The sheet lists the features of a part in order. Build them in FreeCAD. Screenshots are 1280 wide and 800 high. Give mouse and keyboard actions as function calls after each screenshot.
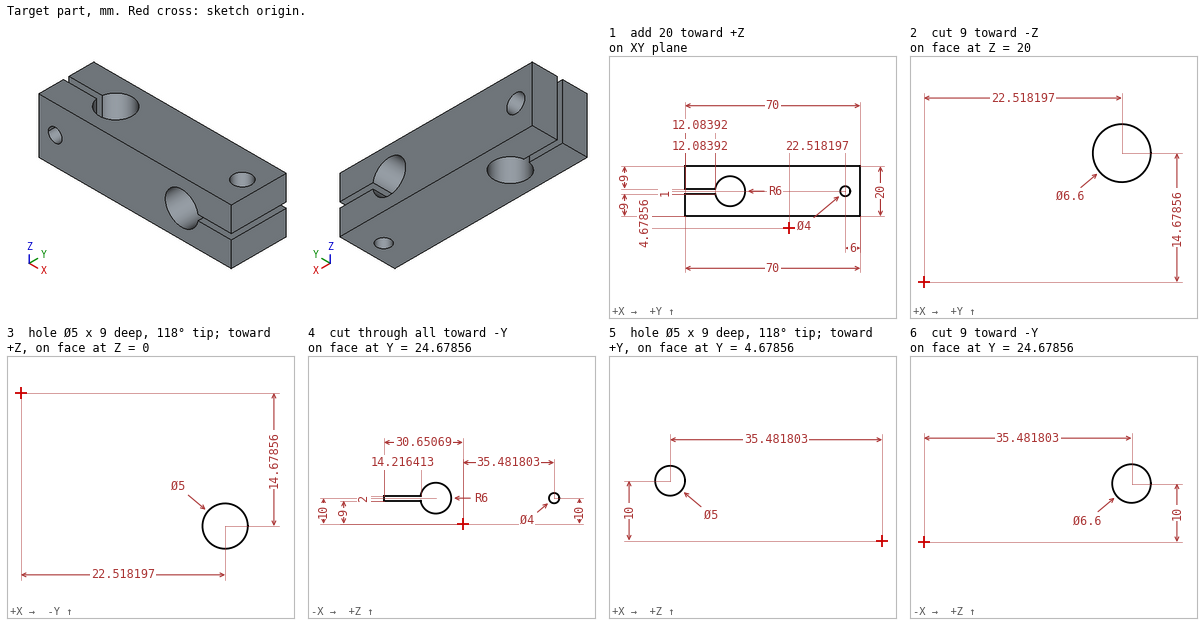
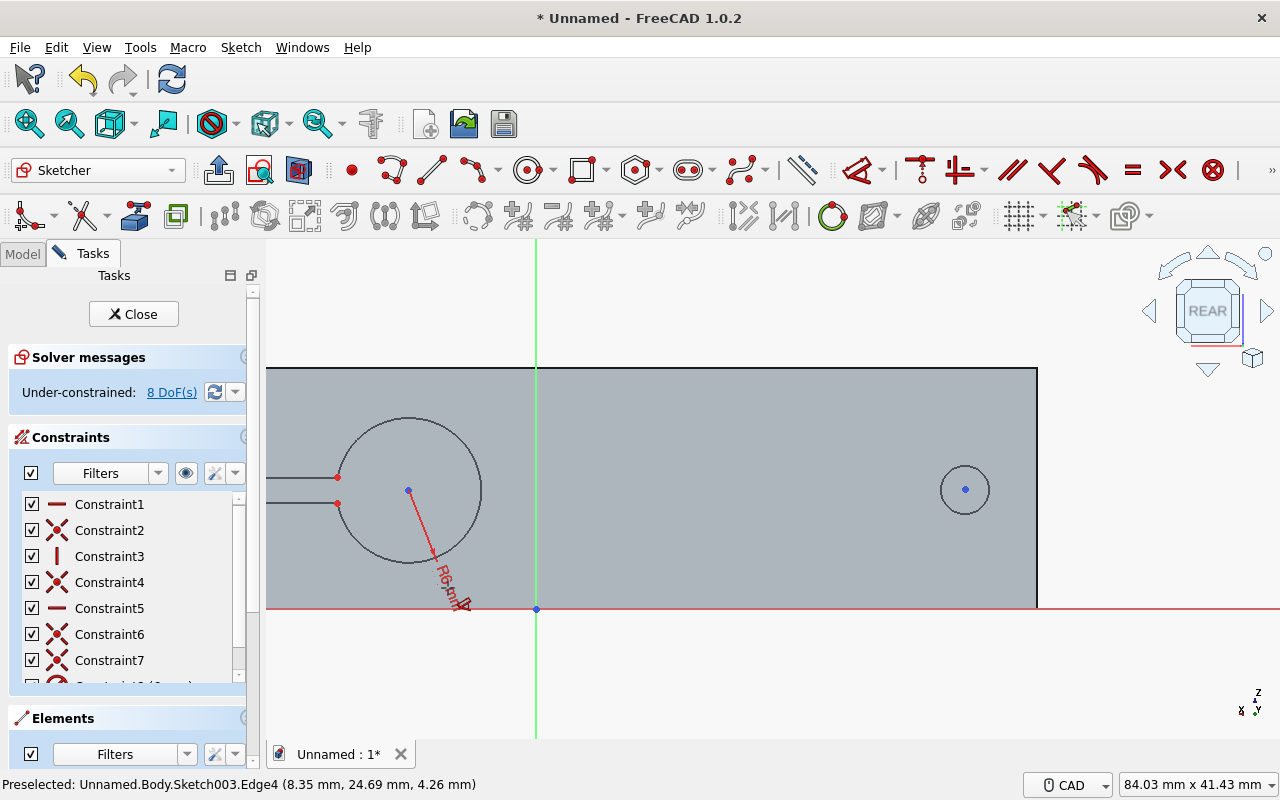
click(982, 473)
click(1005, 450)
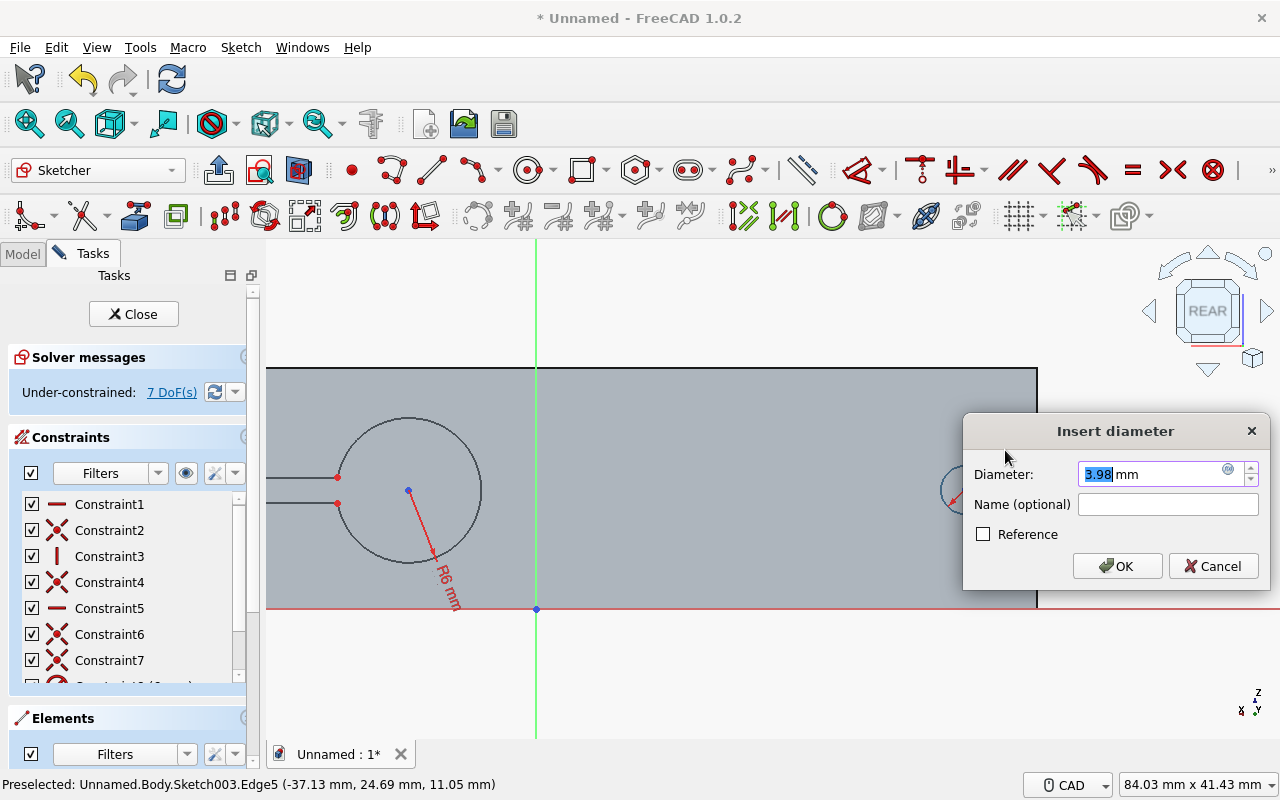
text(4)
key(Return)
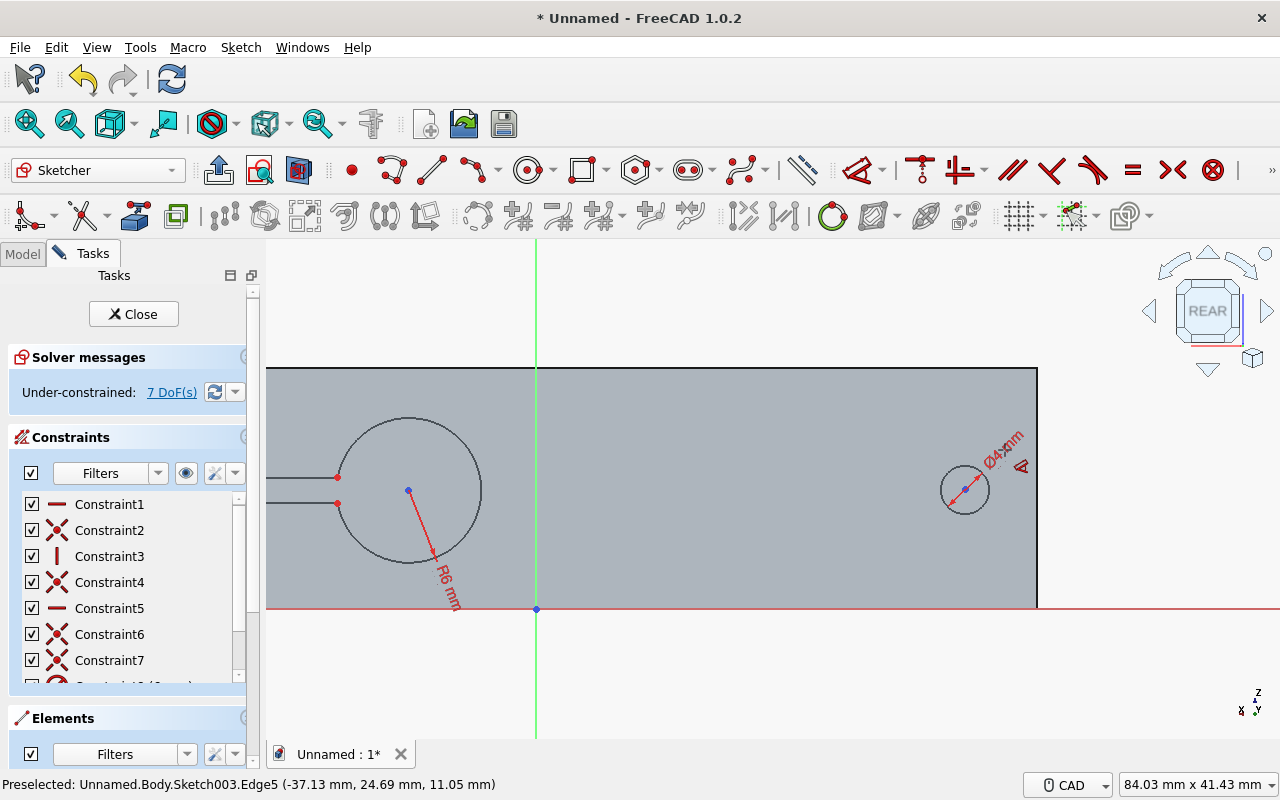
scroll(963, 392, down, 2)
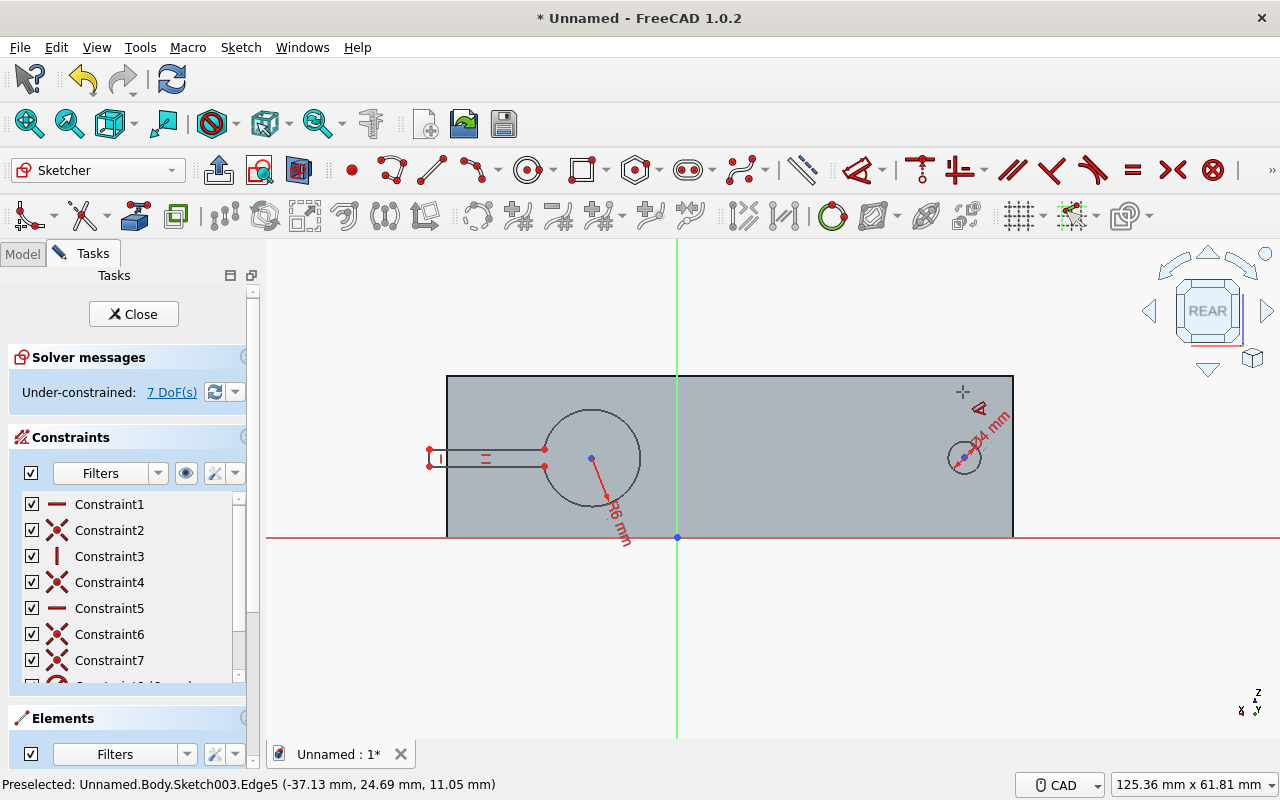
scroll(429, 456, up, 5)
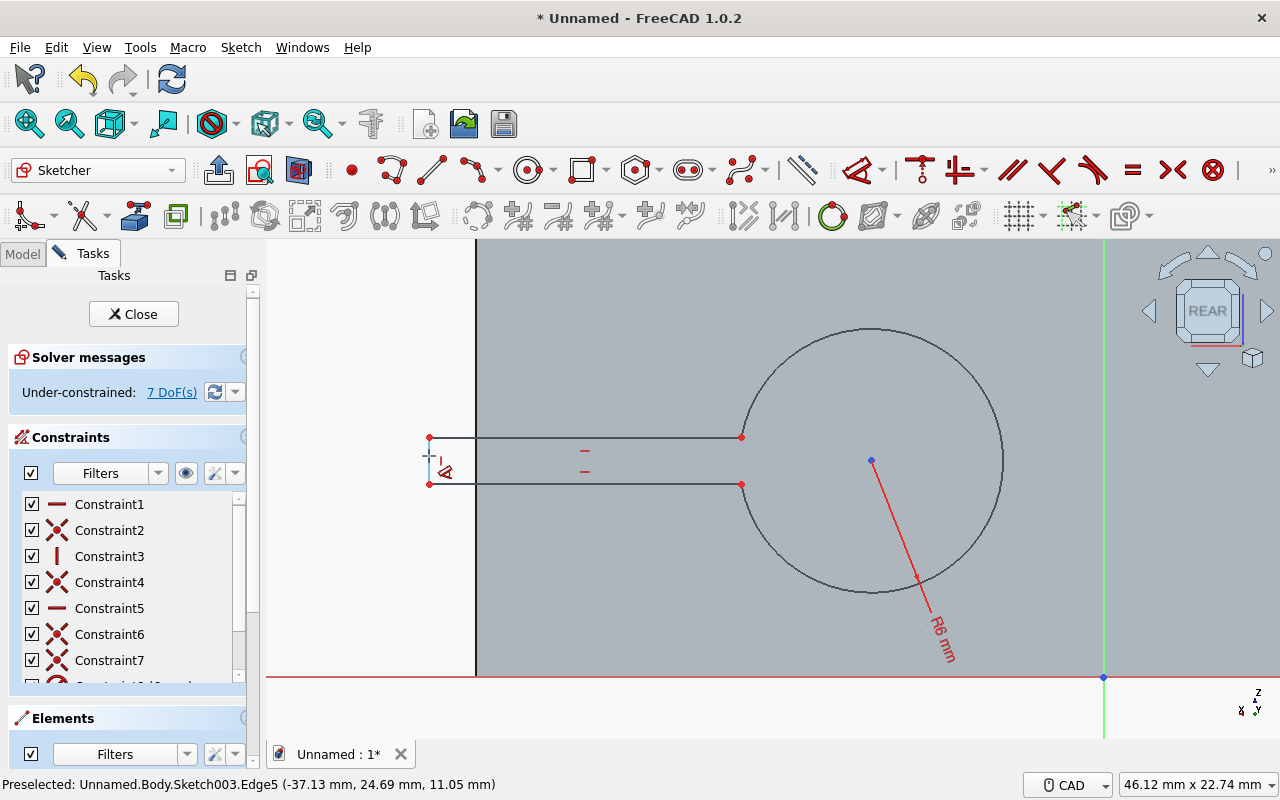
click(429, 456)
click(395, 461)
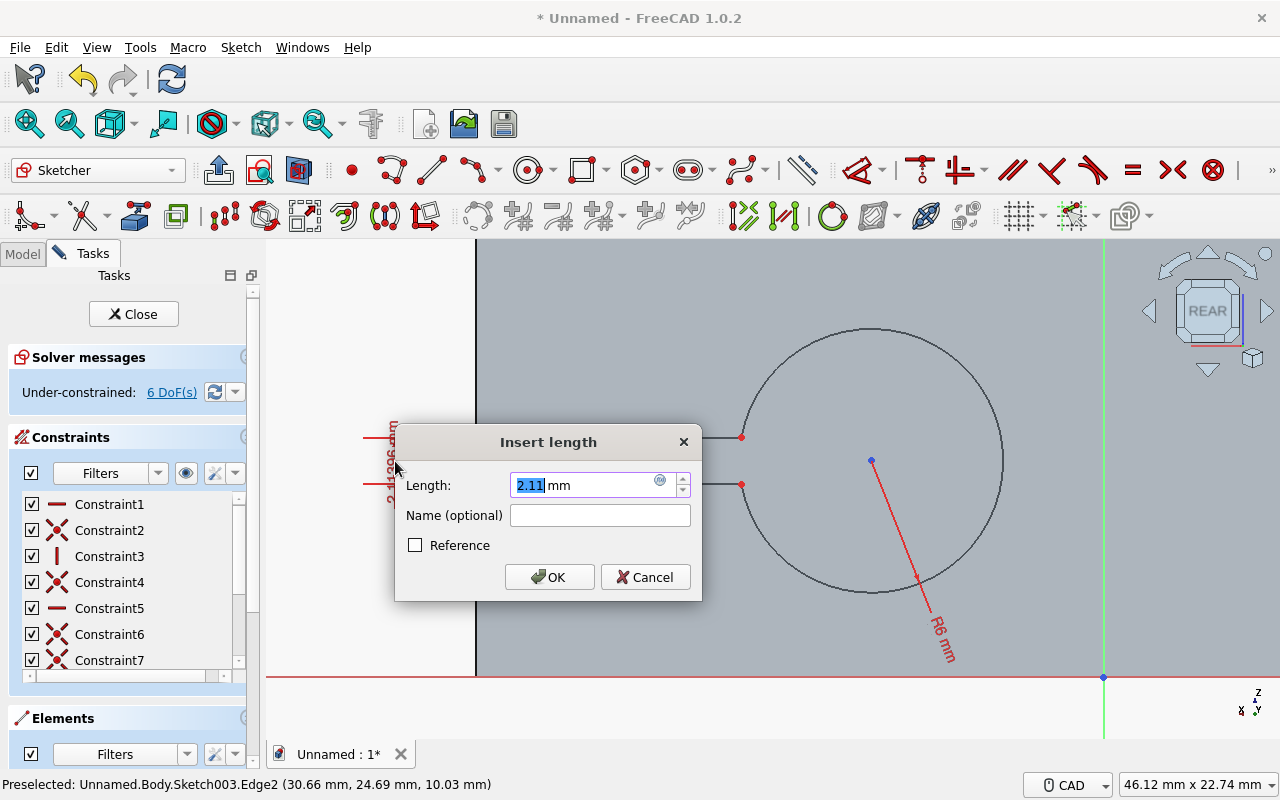
text(2)
key(Return)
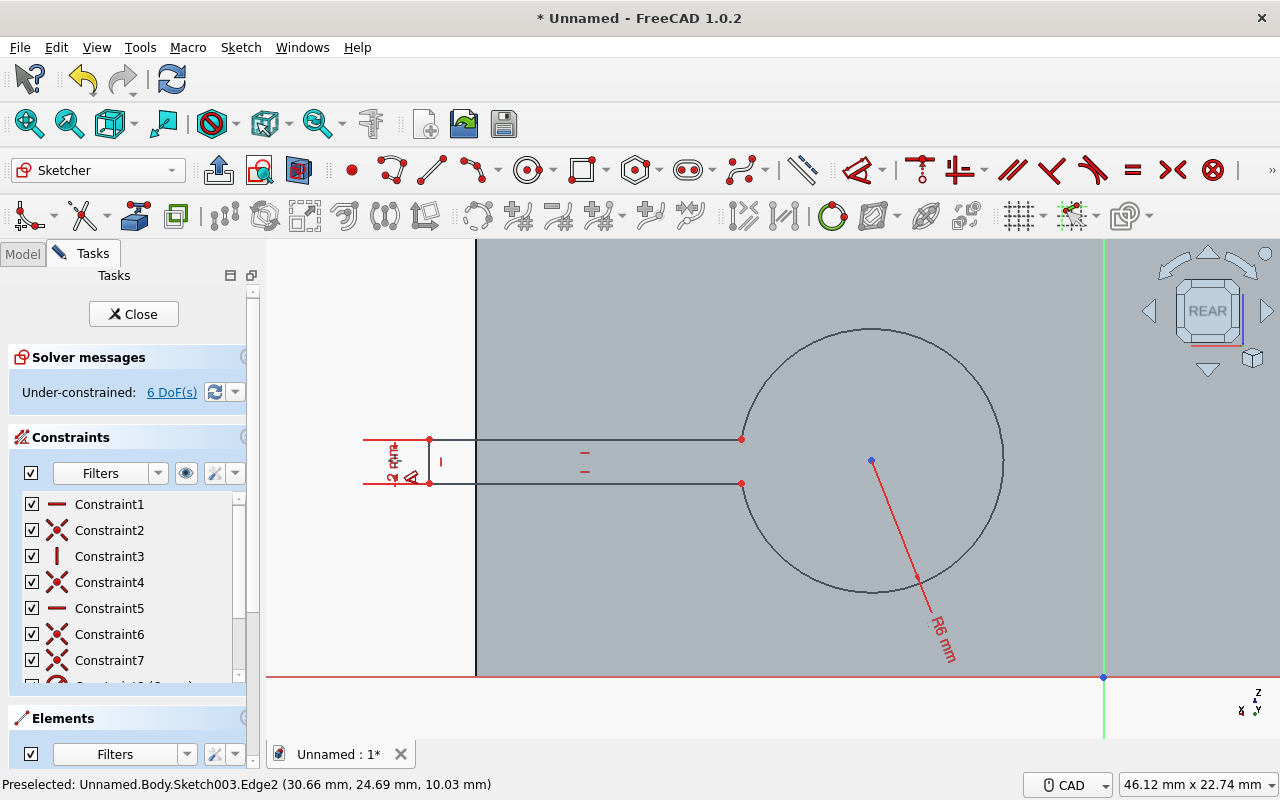
click(429, 484)
click(395, 581)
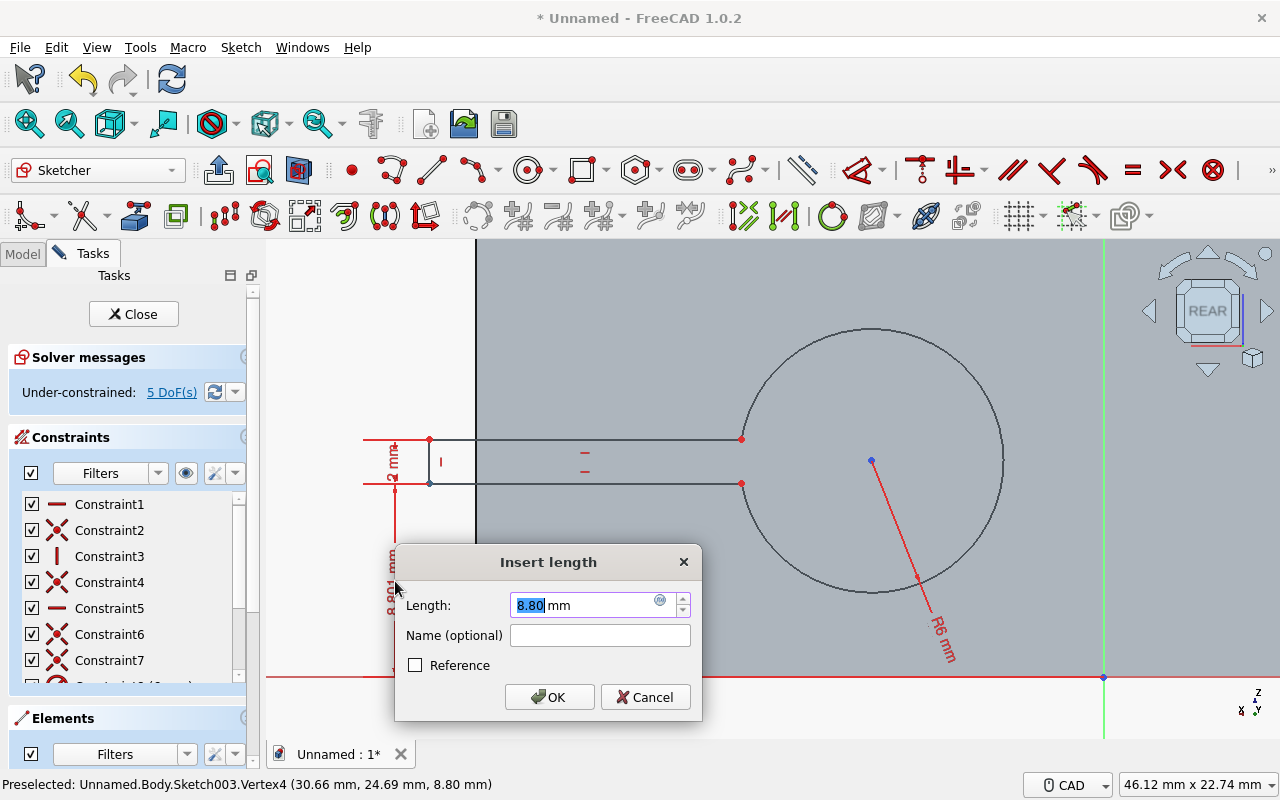
text(9)
key(Return)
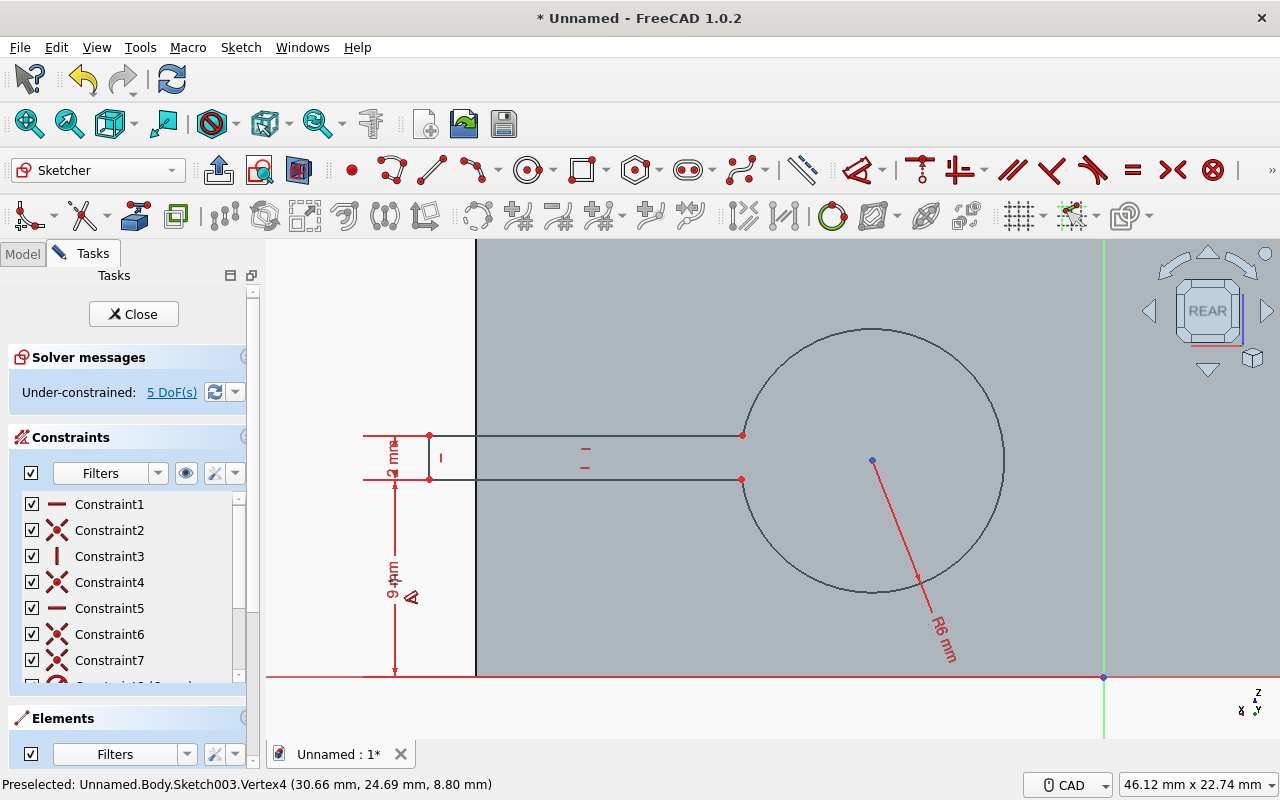
scroll(429, 456, down, 5)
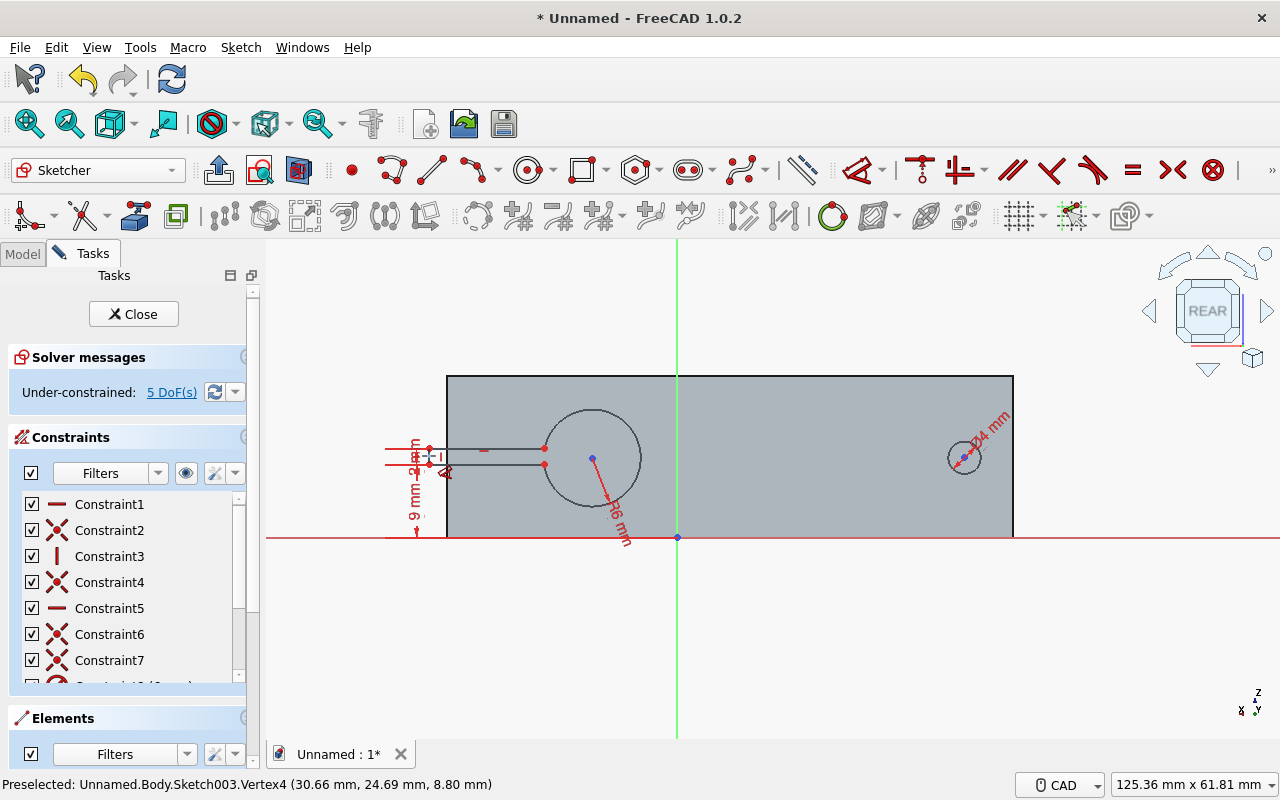
click(965, 458)
click(999, 498)